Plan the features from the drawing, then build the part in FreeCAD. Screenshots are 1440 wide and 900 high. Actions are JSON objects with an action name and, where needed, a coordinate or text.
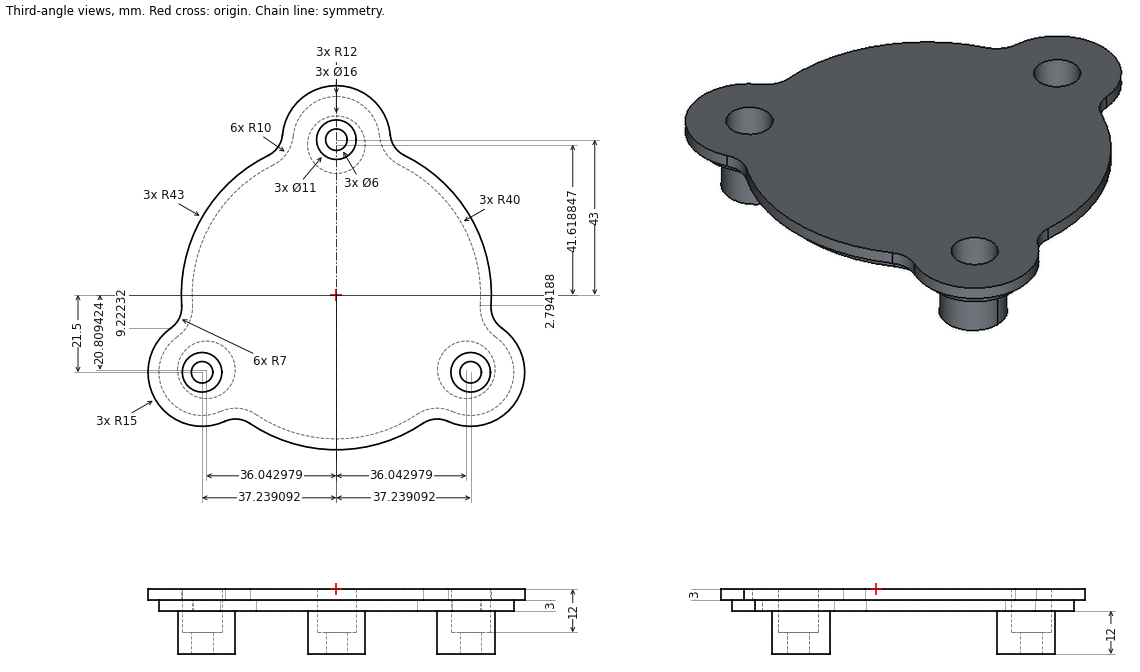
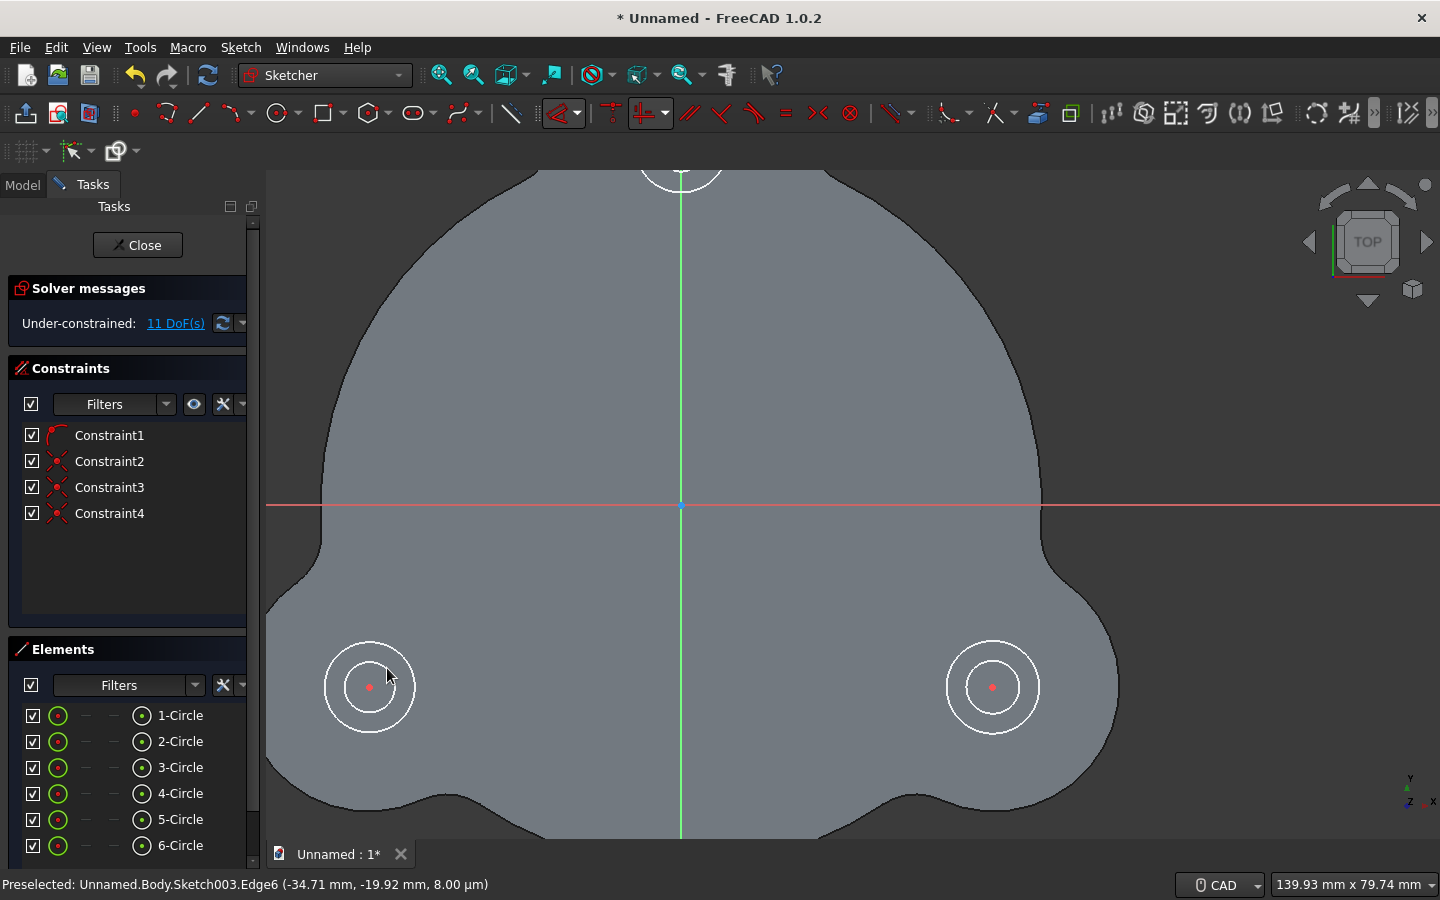
{"action": "scroll", "coordinate": [994, 686], "scroll_direction": "down", "scroll_amount": 2}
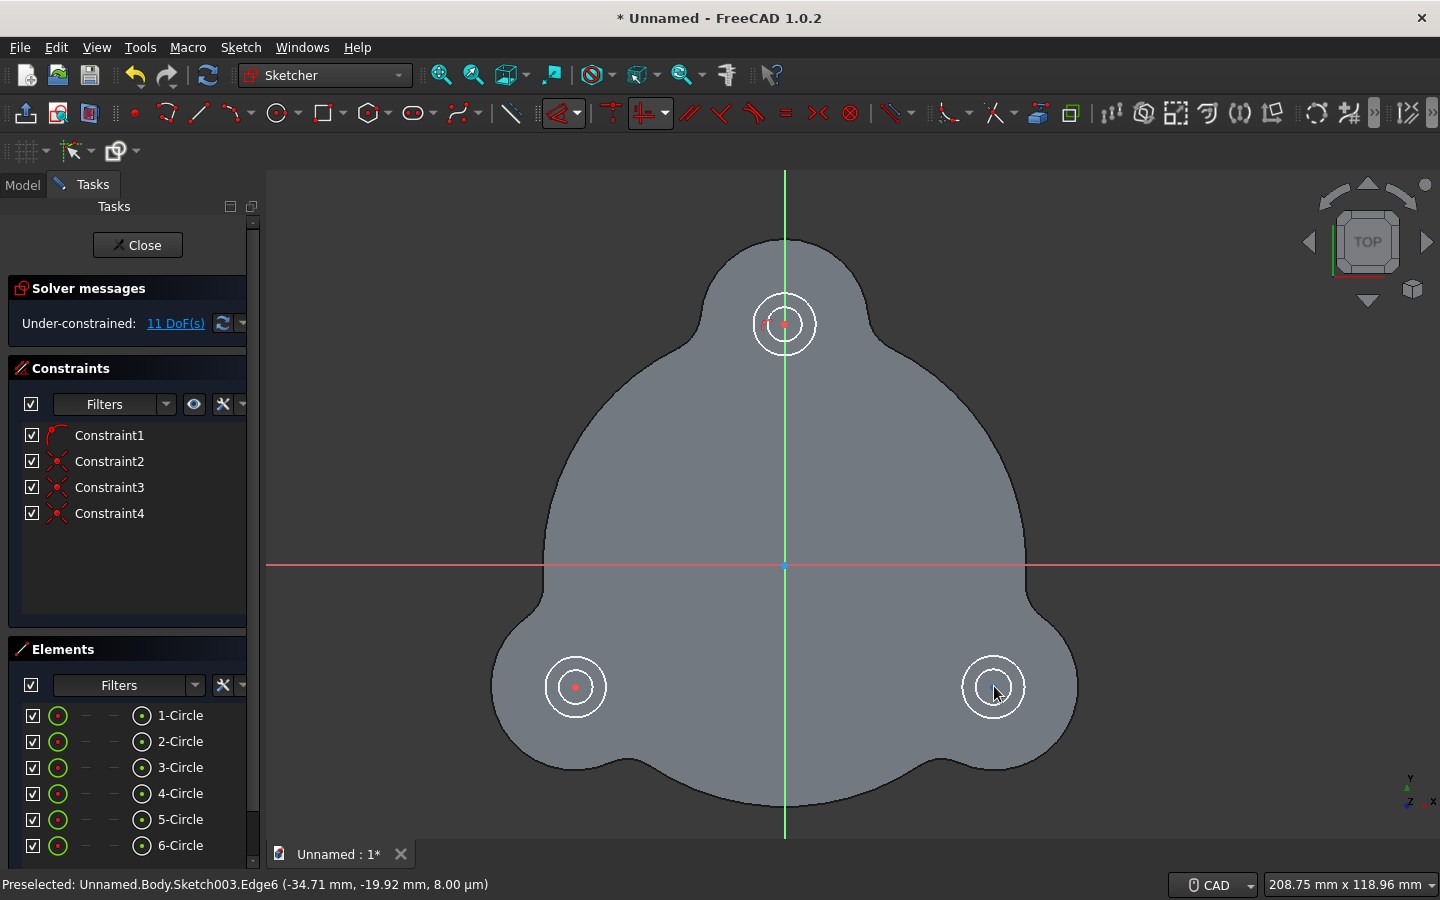
{"action": "left_click", "coordinate": [807, 302]}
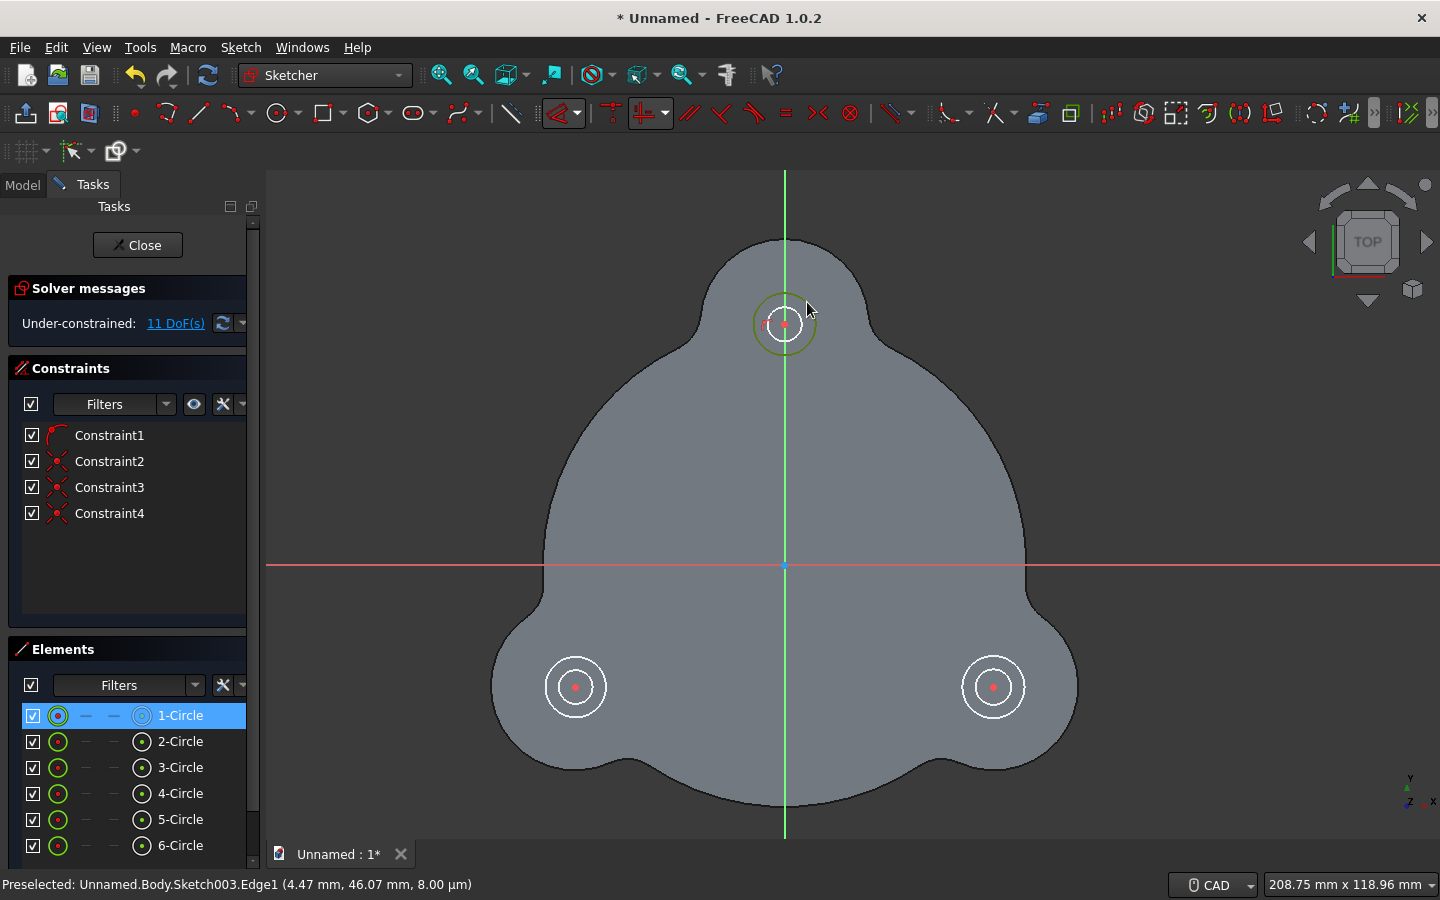
{"action": "left_click", "coordinate": [1015, 665]}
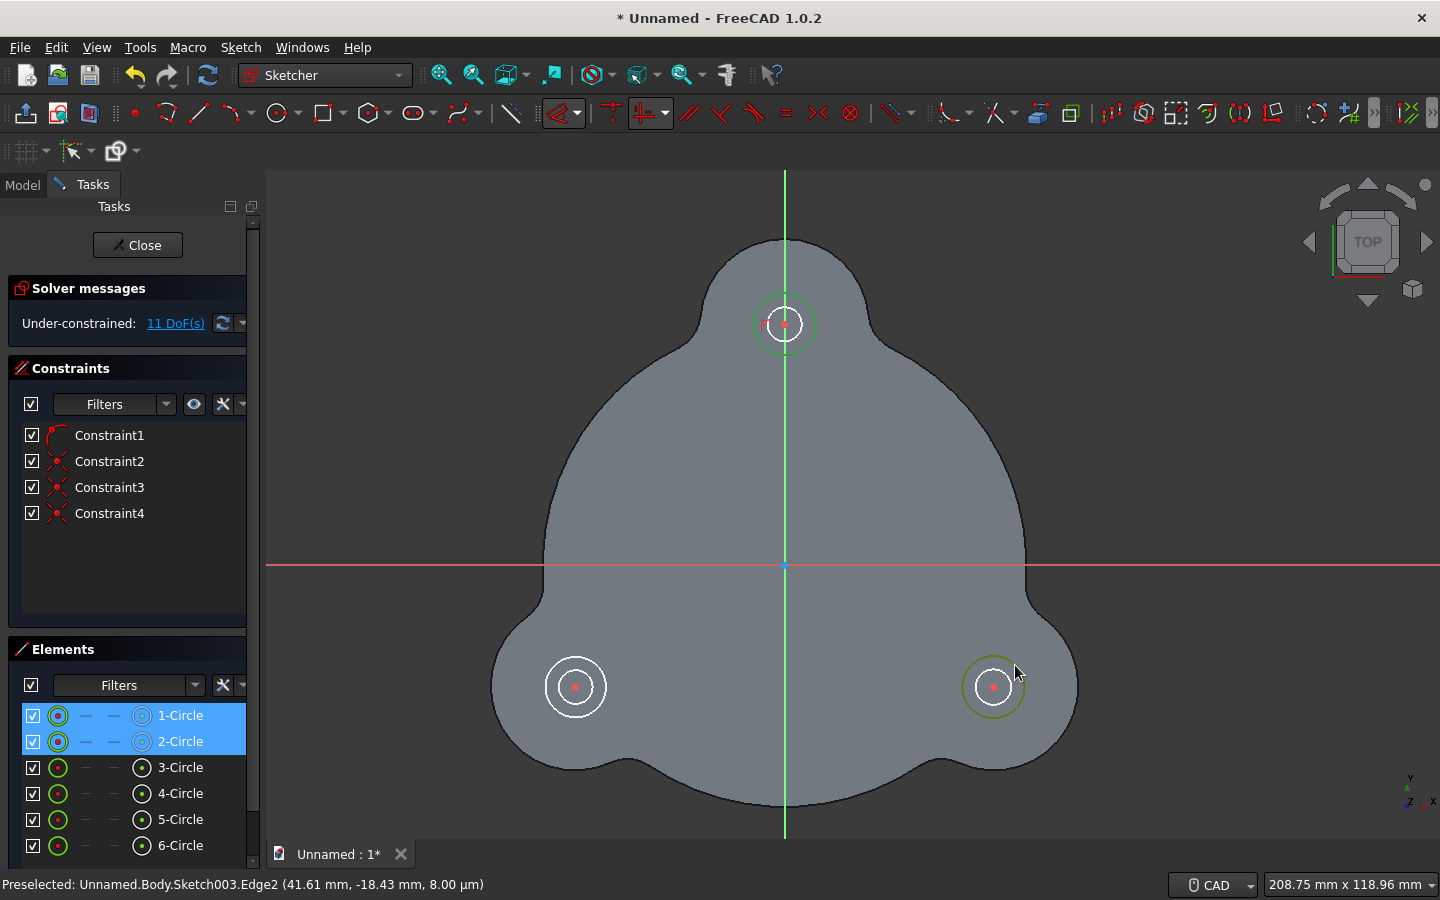
{"action": "left_click", "coordinate": [597, 666]}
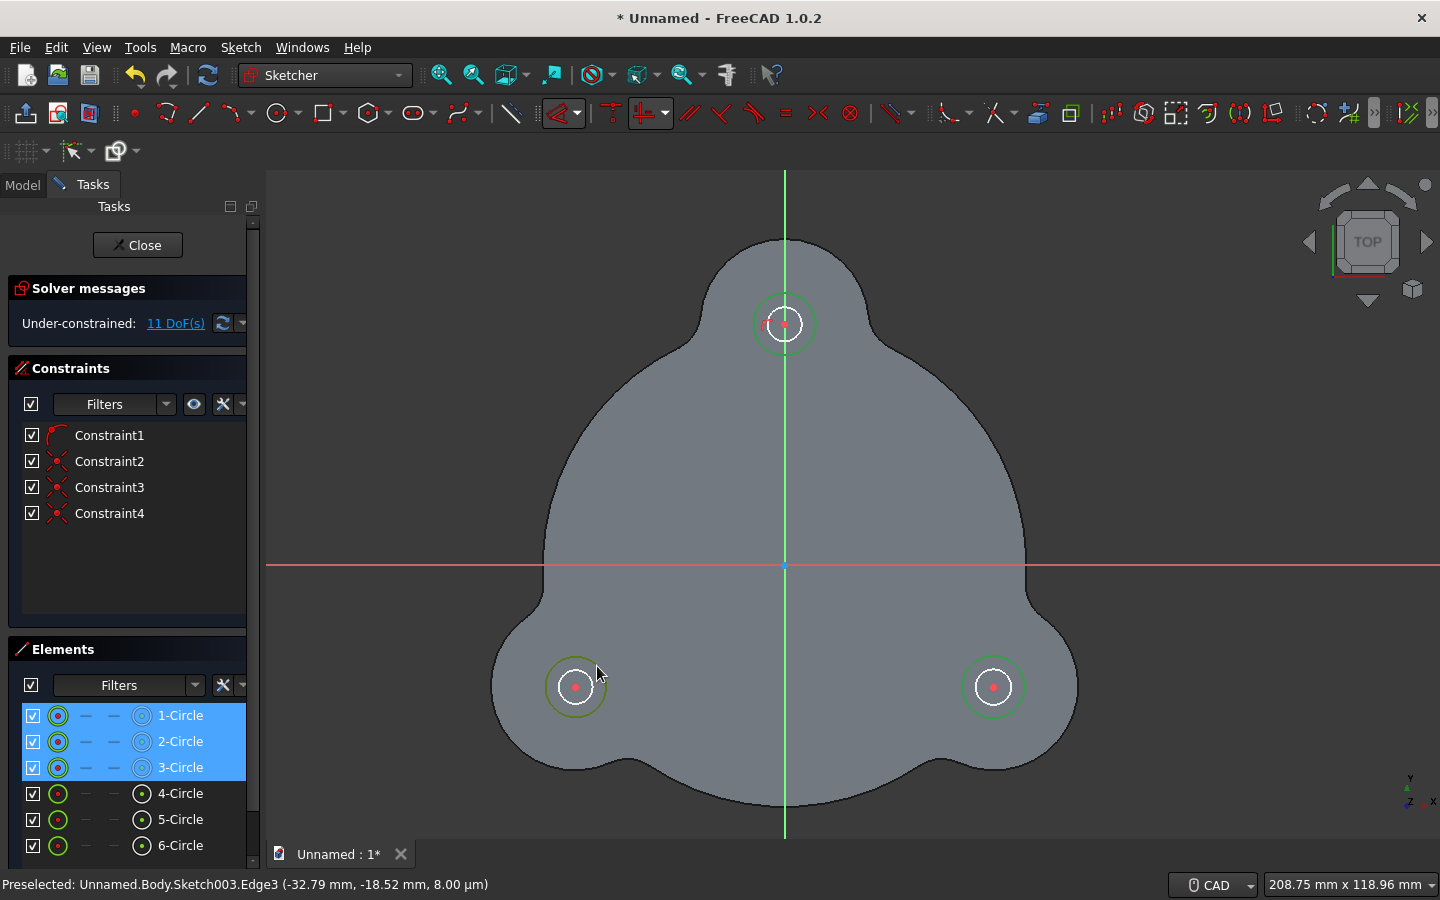
{"action": "left_click", "coordinate": [786, 114]}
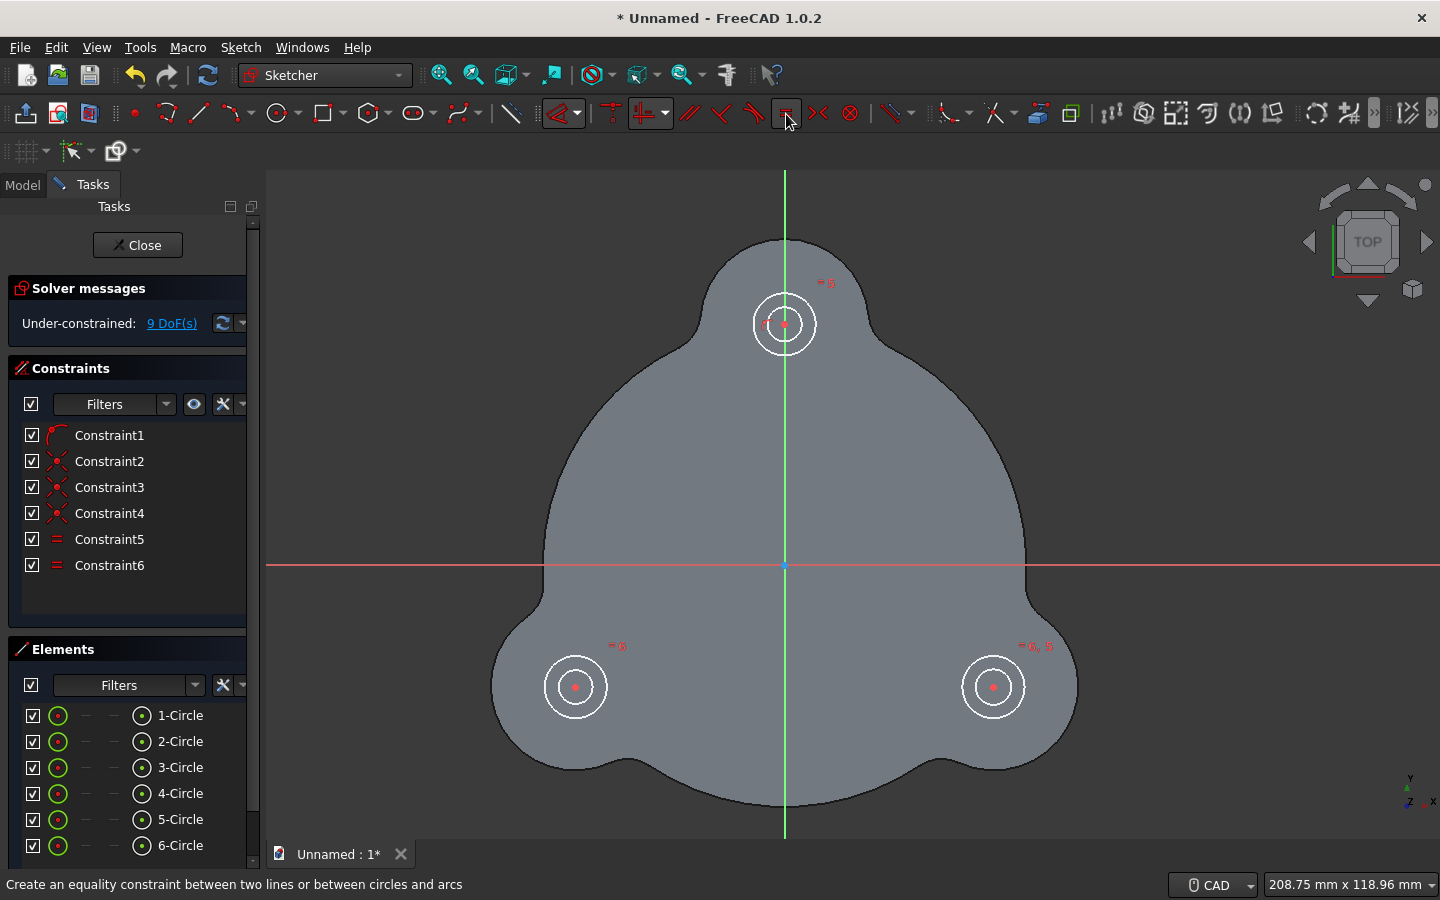
{"action": "left_click", "coordinate": [797, 312]}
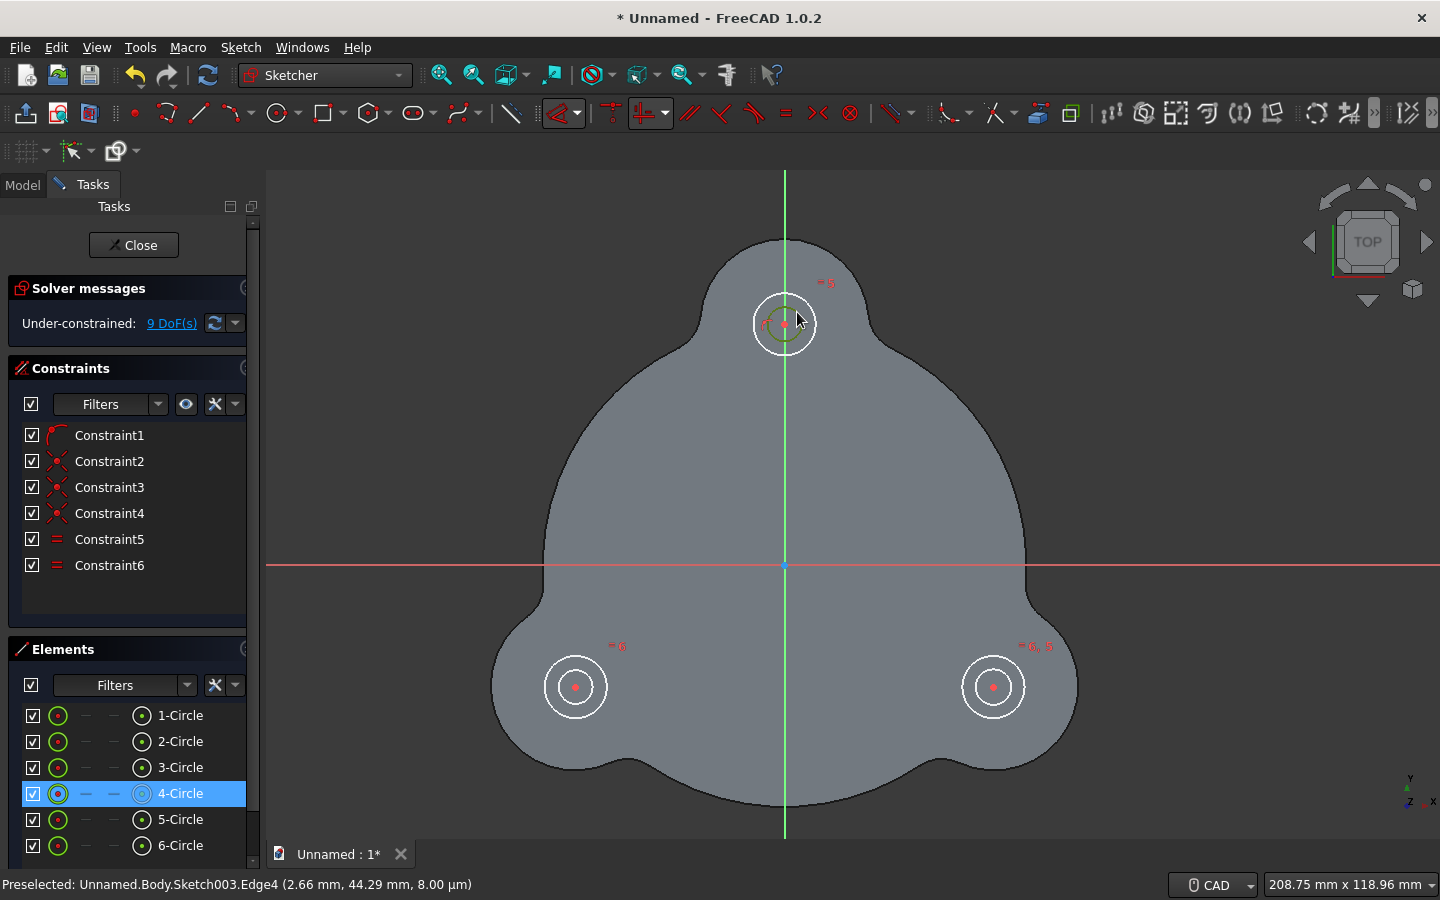
{"action": "left_click", "coordinate": [1006, 675]}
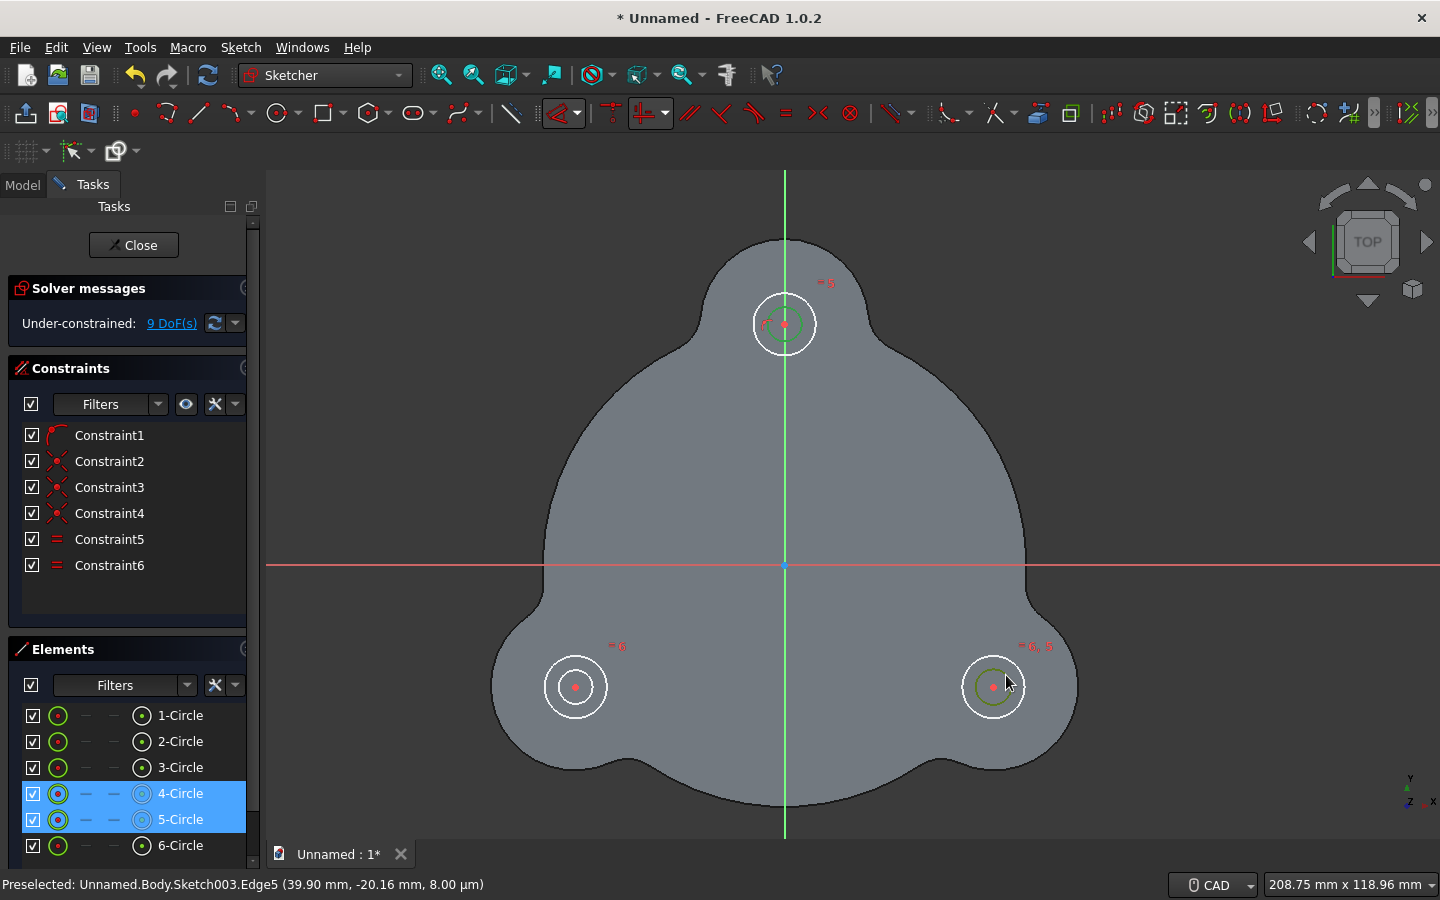
{"action": "left_click", "coordinate": [588, 675]}